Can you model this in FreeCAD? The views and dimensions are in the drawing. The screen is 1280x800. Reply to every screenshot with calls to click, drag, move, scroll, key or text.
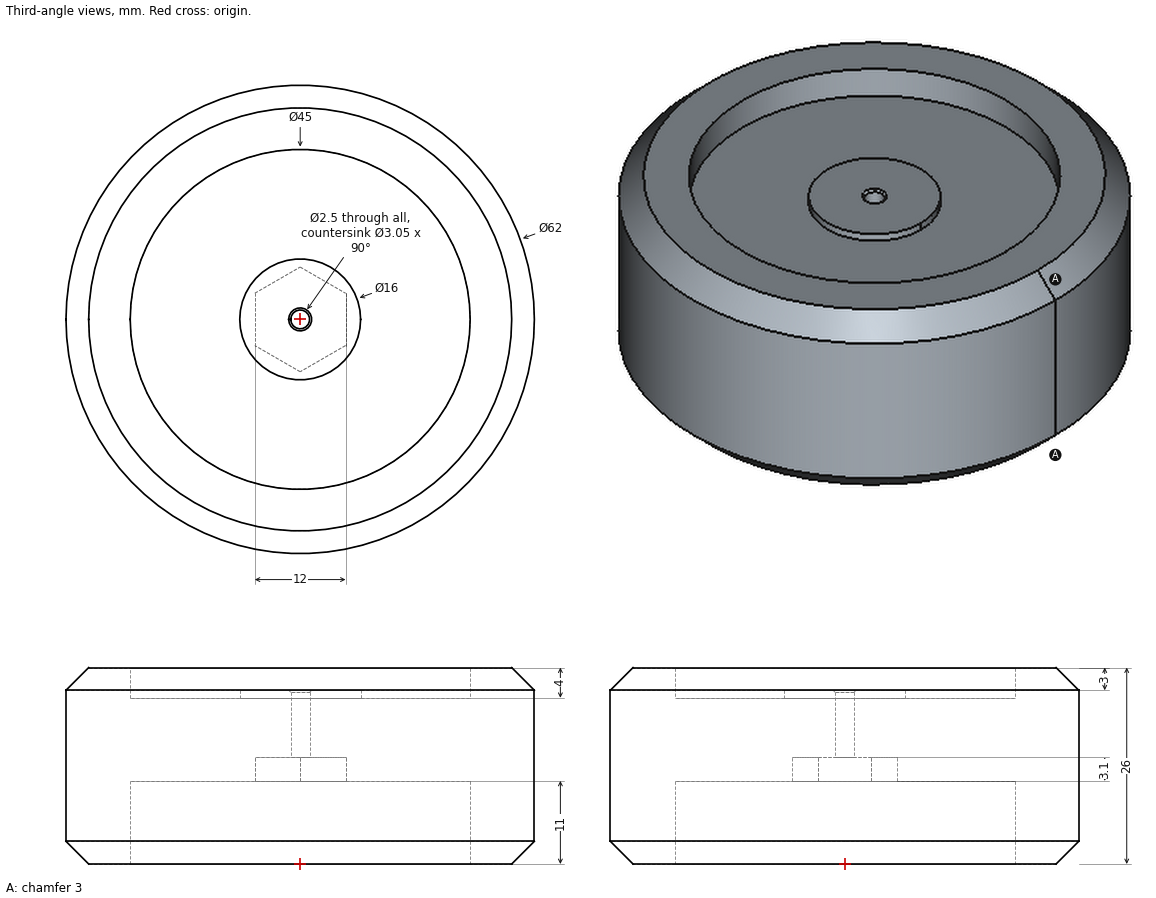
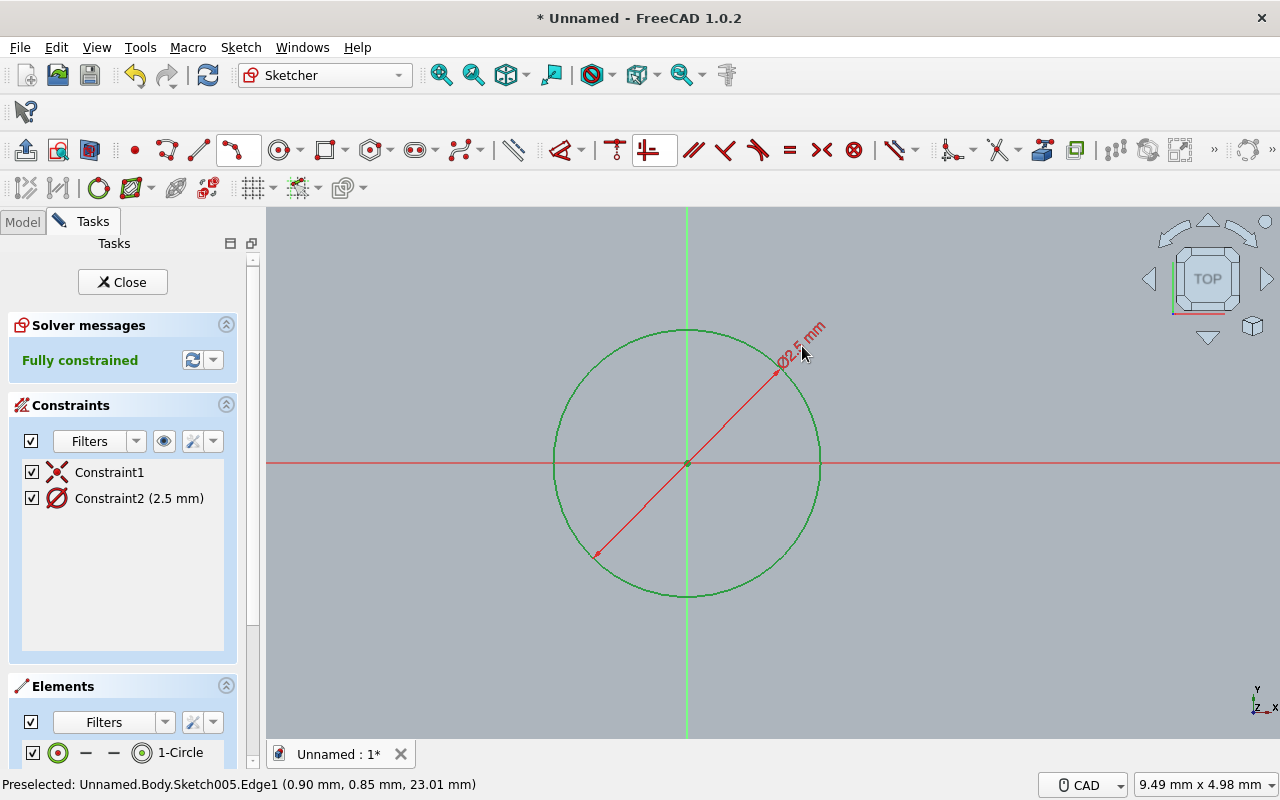
click(123, 282)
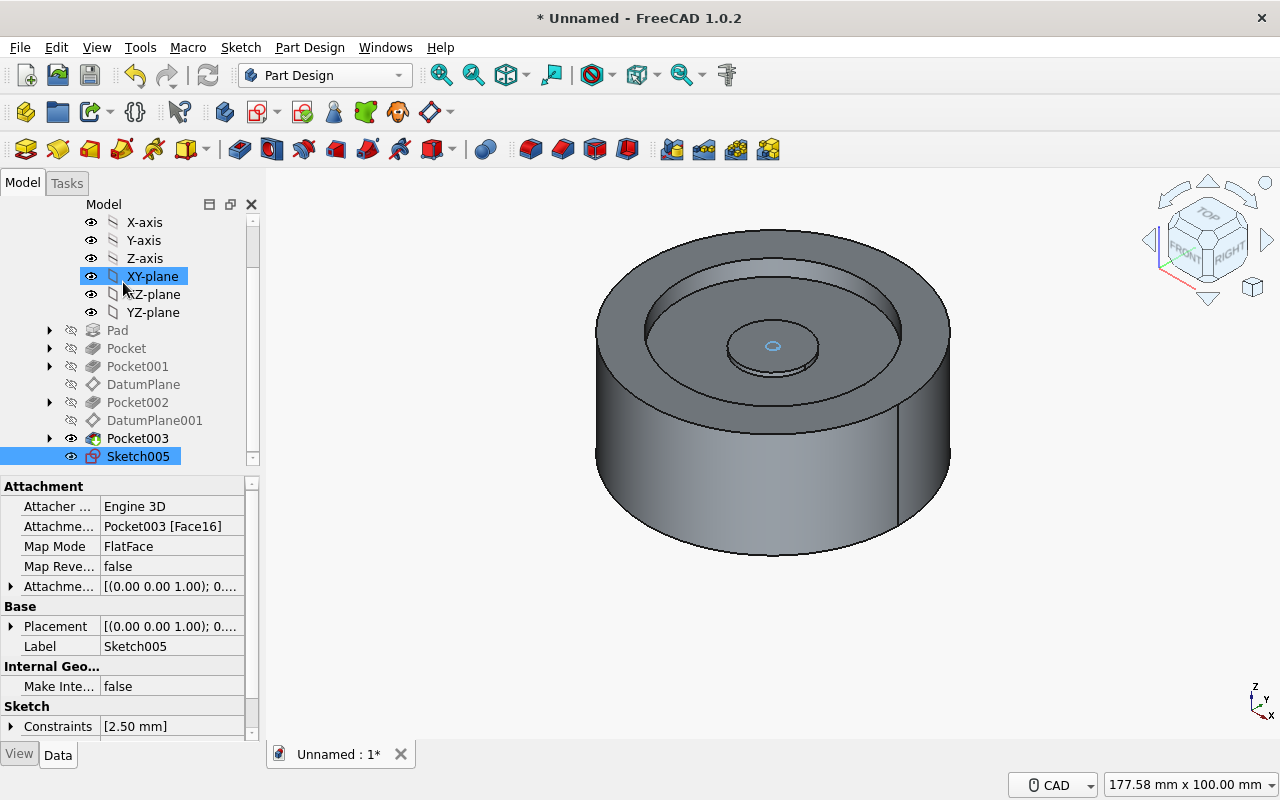
click(272, 150)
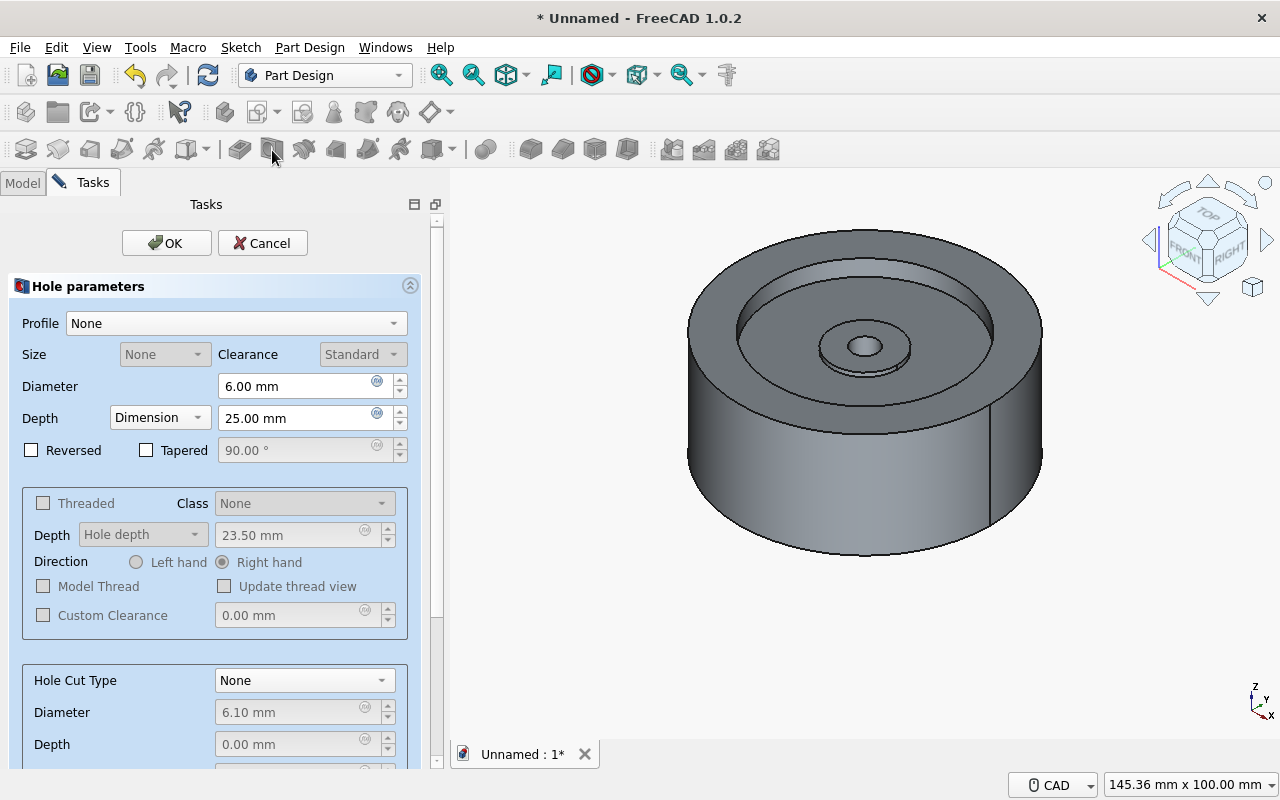
triple_click(305, 386)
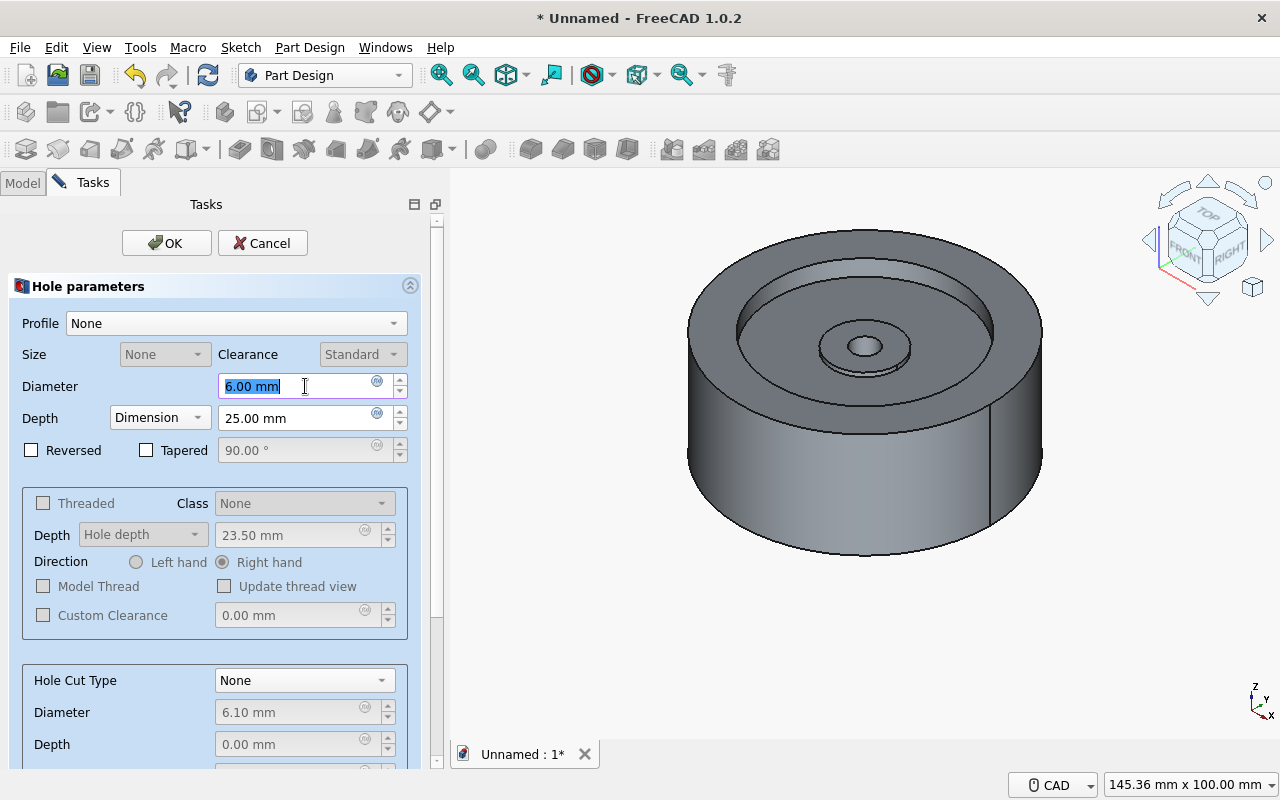
text(2.5)
key(Tab)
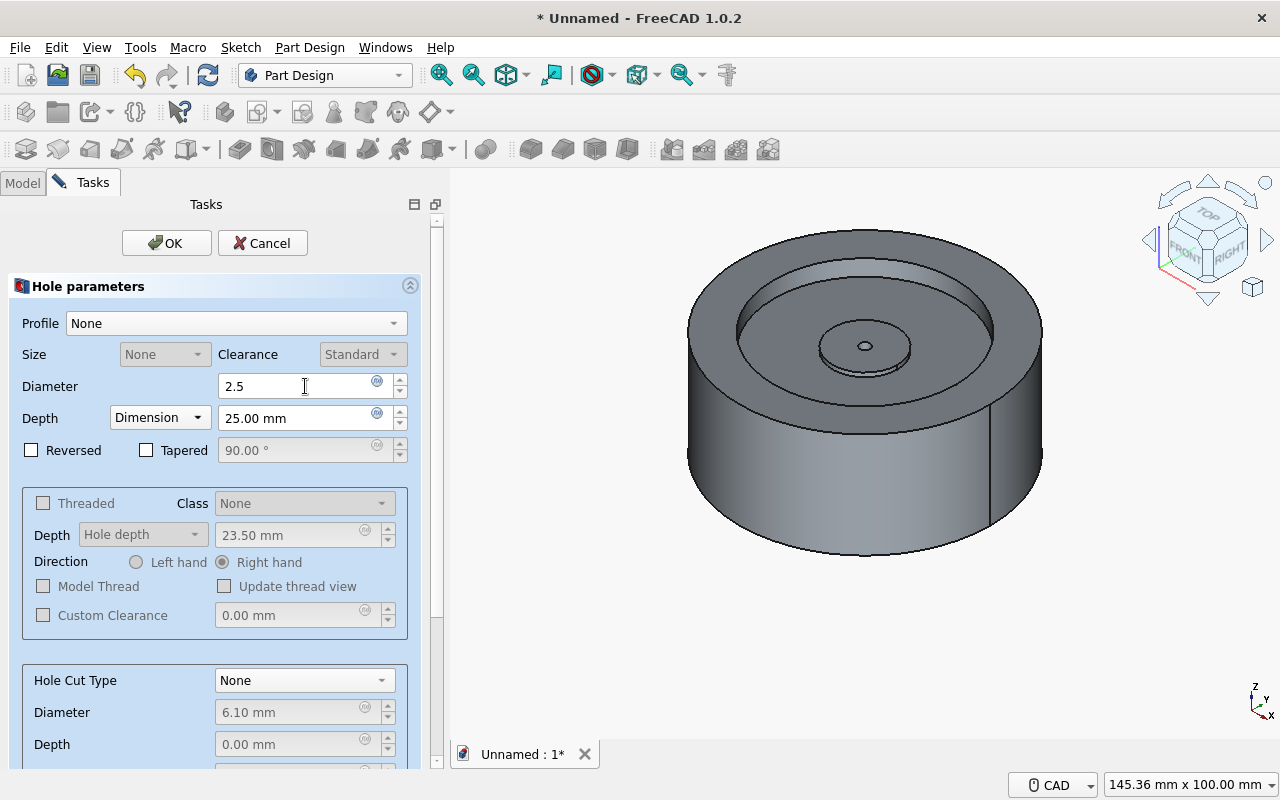
click(161, 418)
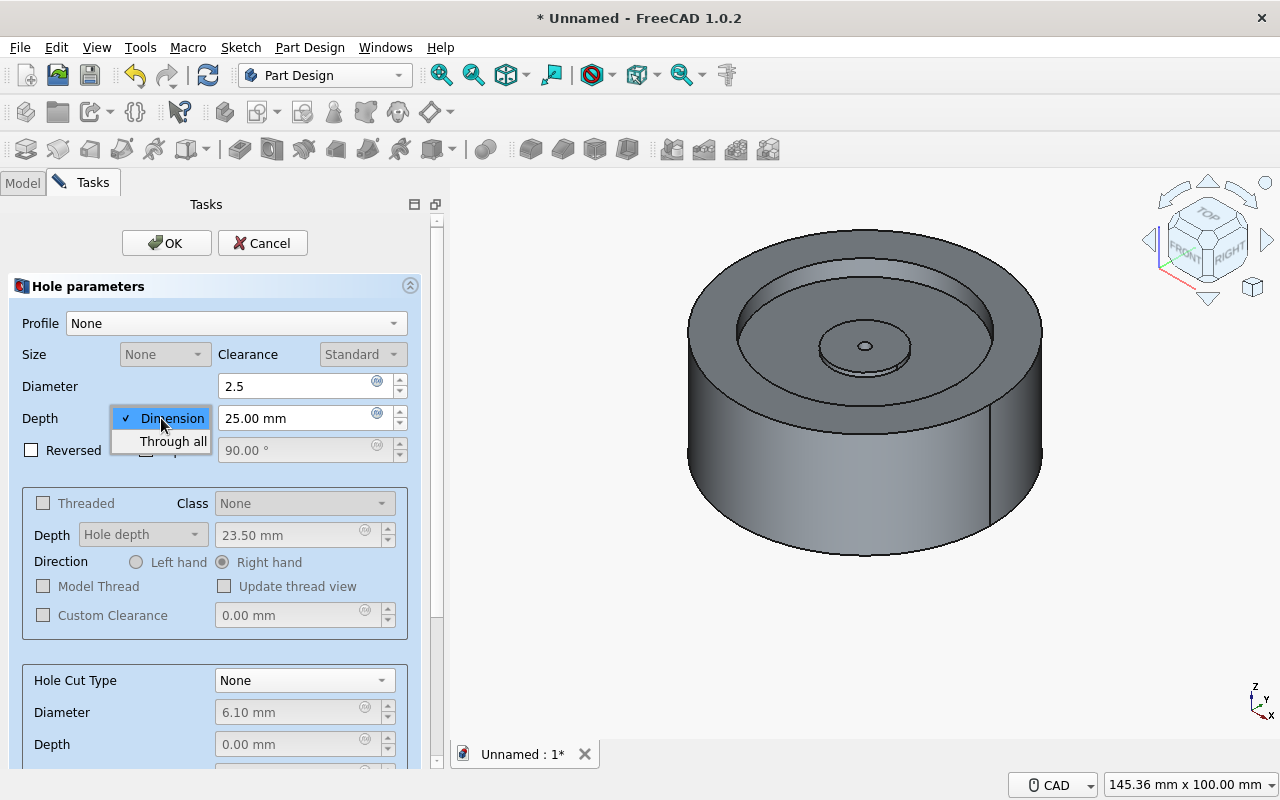
click(160, 442)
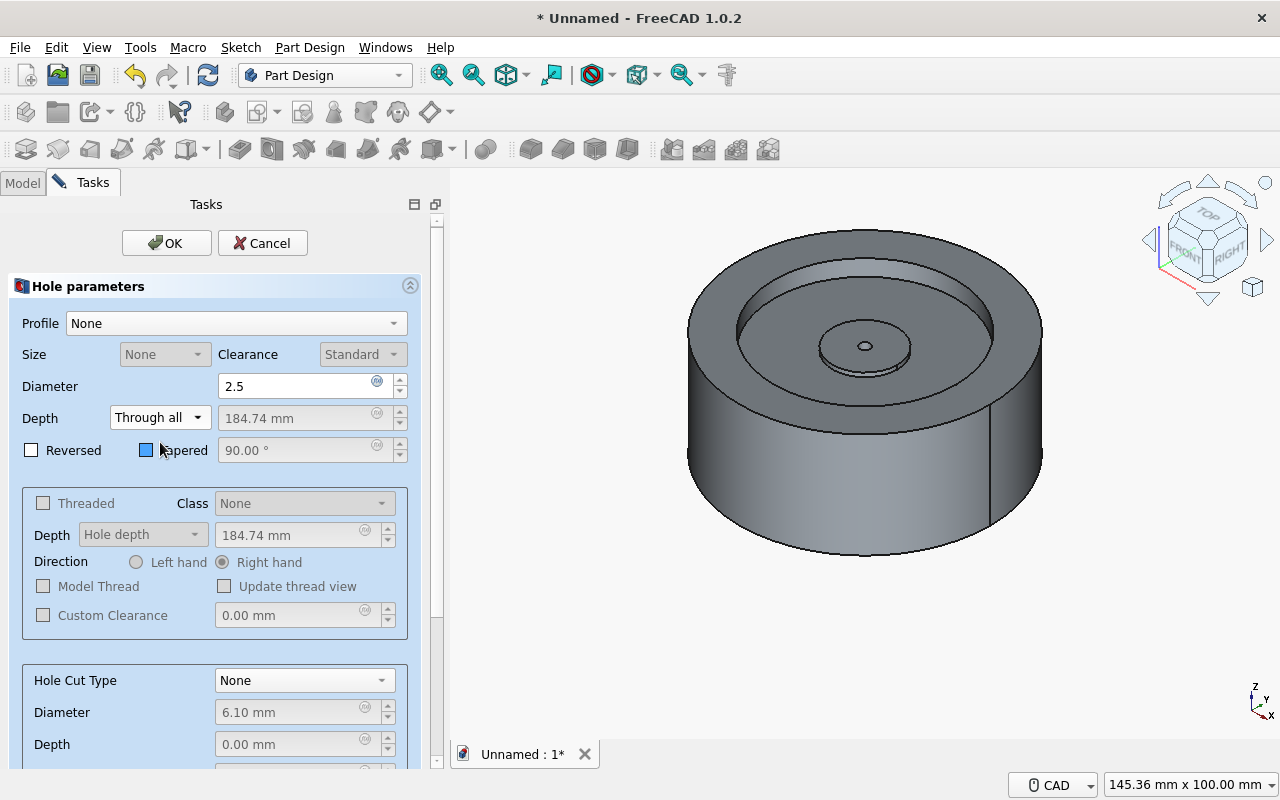
click(306, 680)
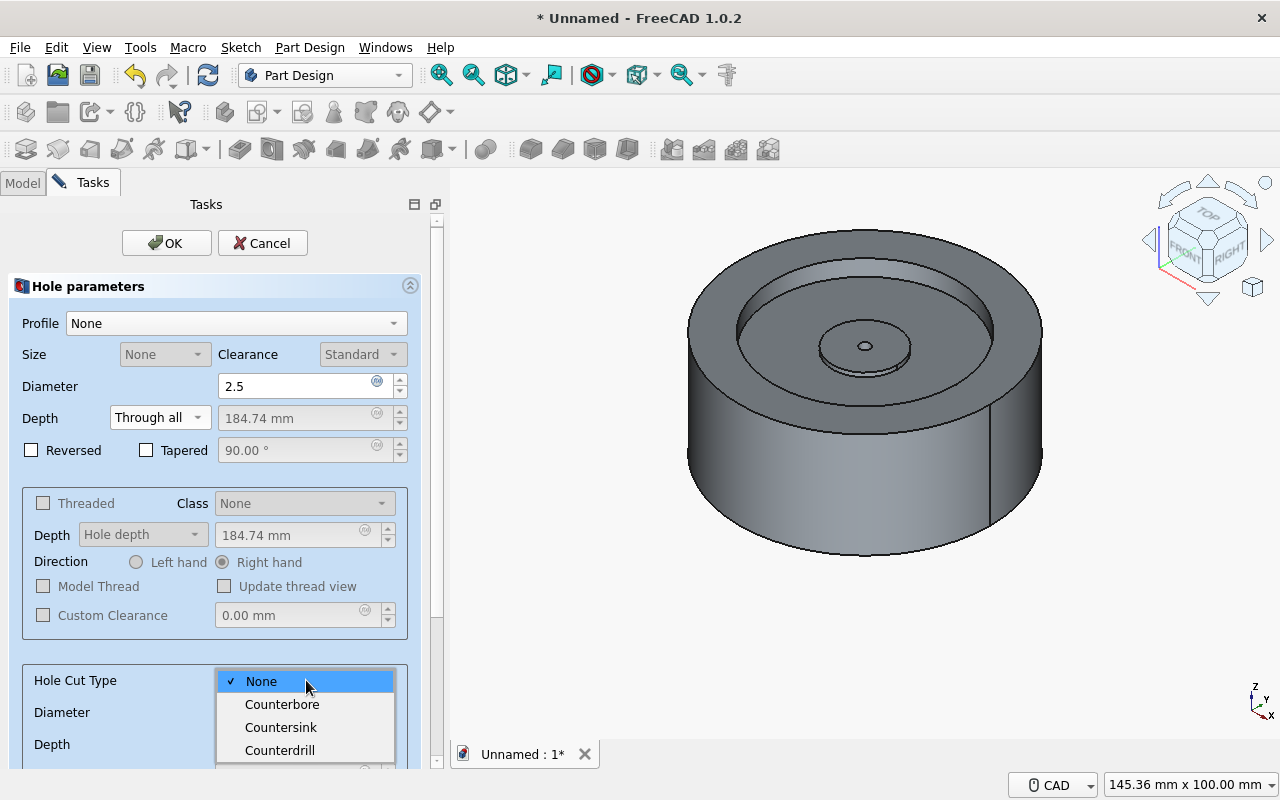
click(304, 728)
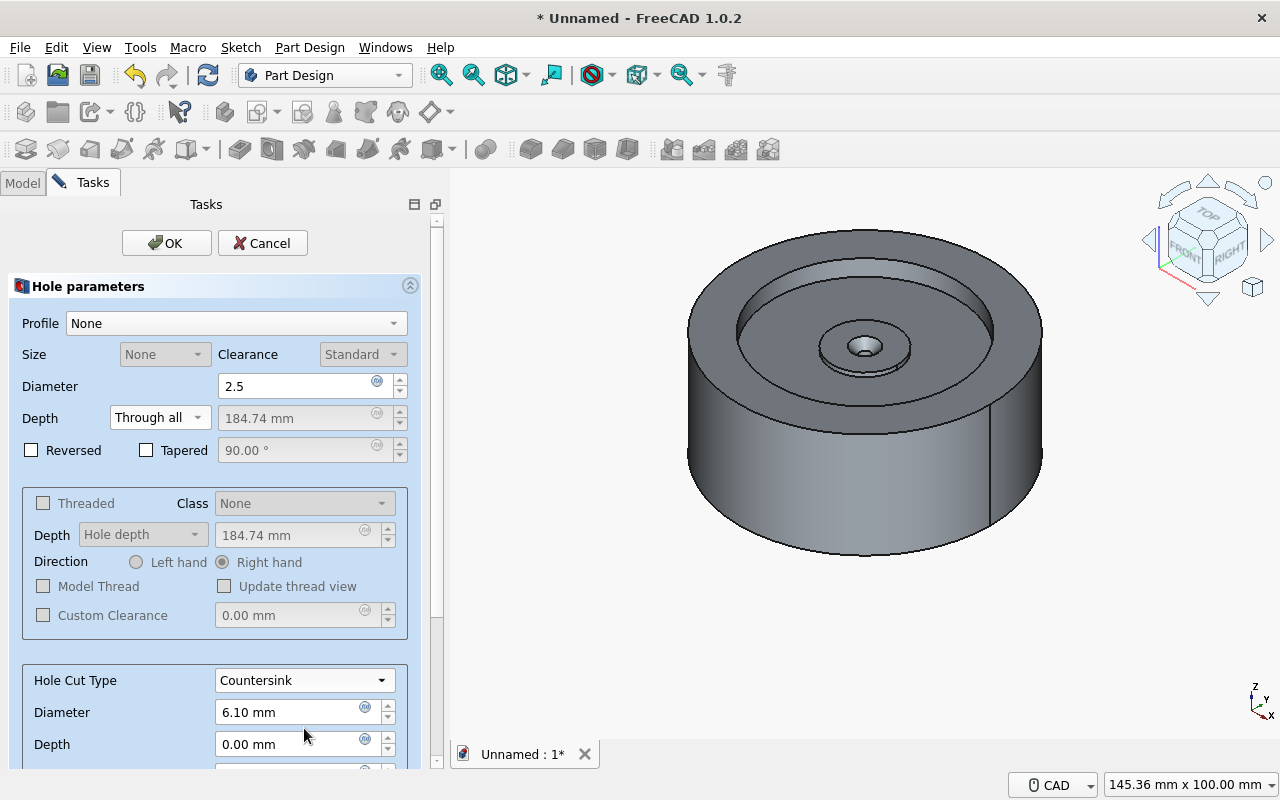
triple_click(298, 712)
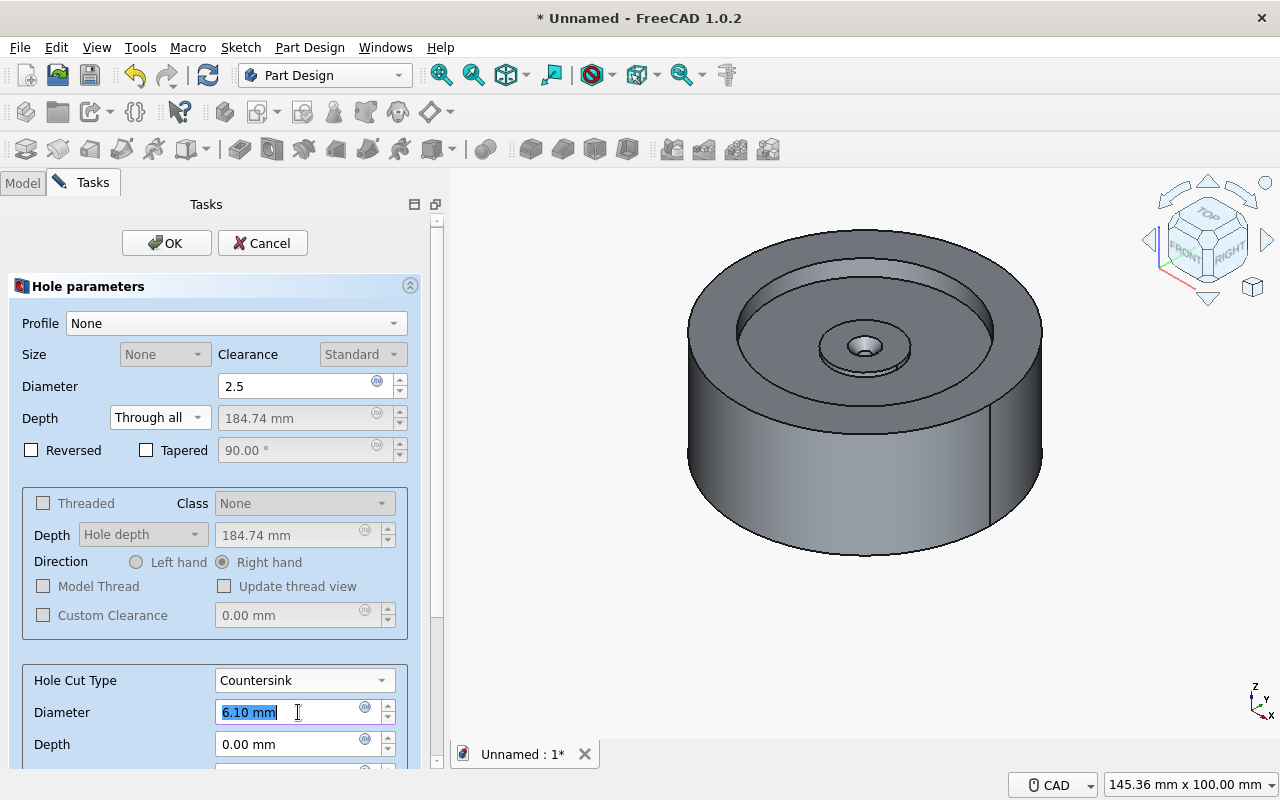
text(3.05)
key(Tab)